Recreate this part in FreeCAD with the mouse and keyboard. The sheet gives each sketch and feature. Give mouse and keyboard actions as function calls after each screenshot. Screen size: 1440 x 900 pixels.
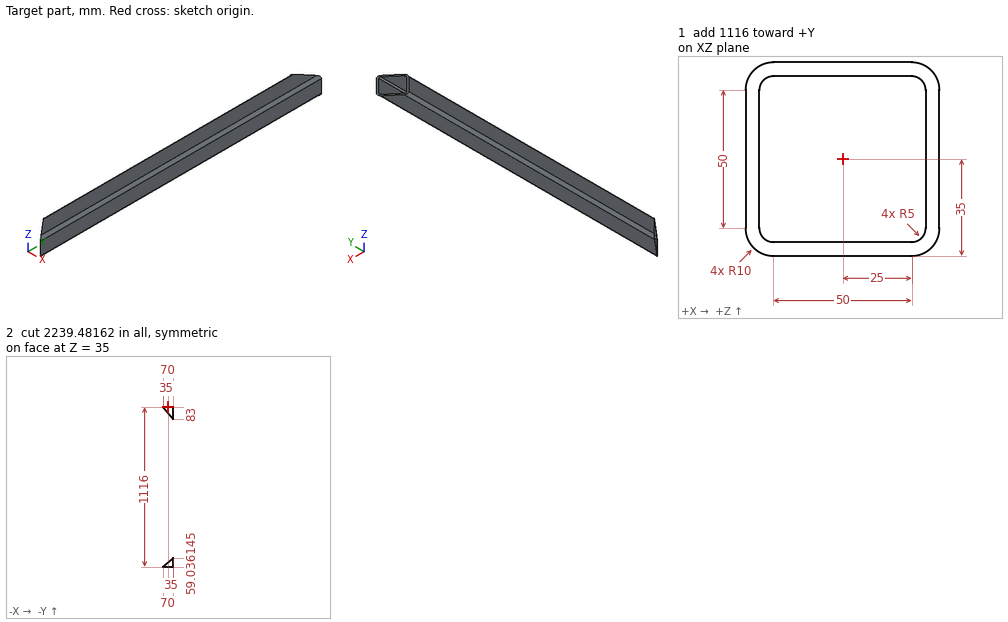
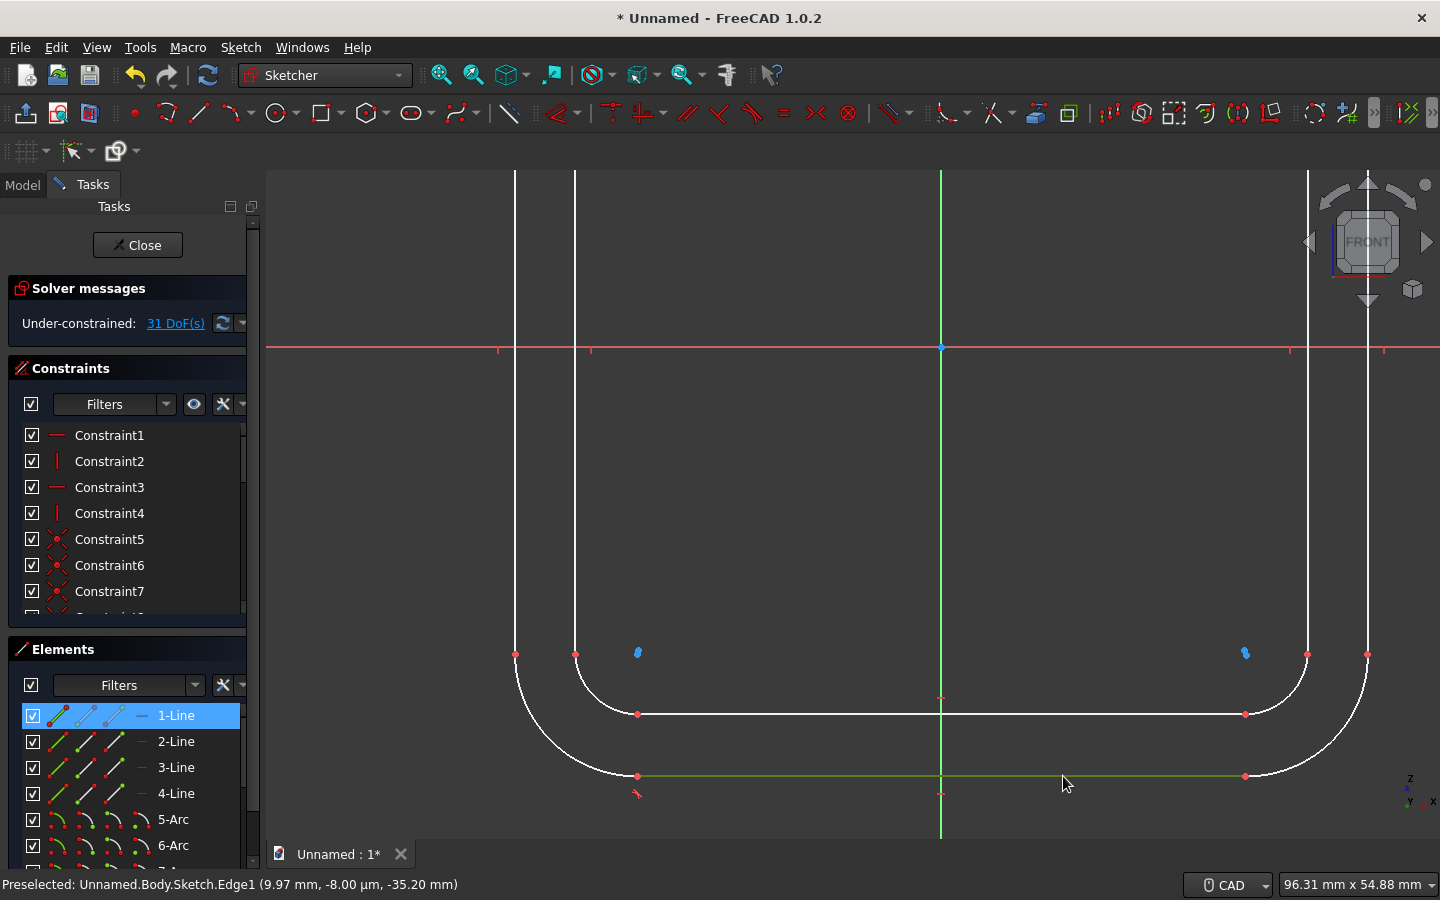
scroll(594, 696, down, 3)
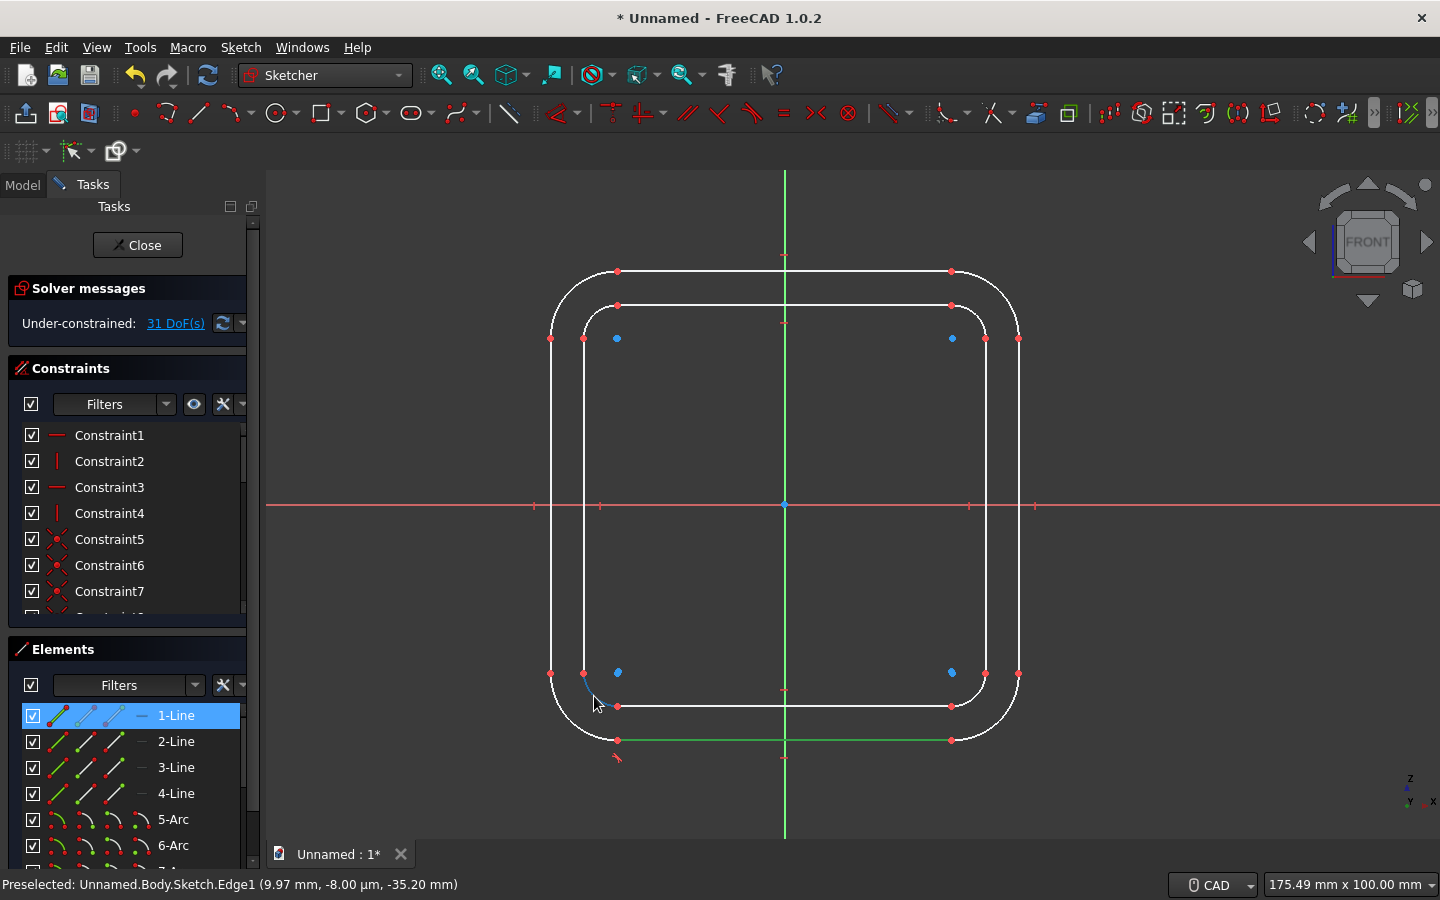
click(982, 733)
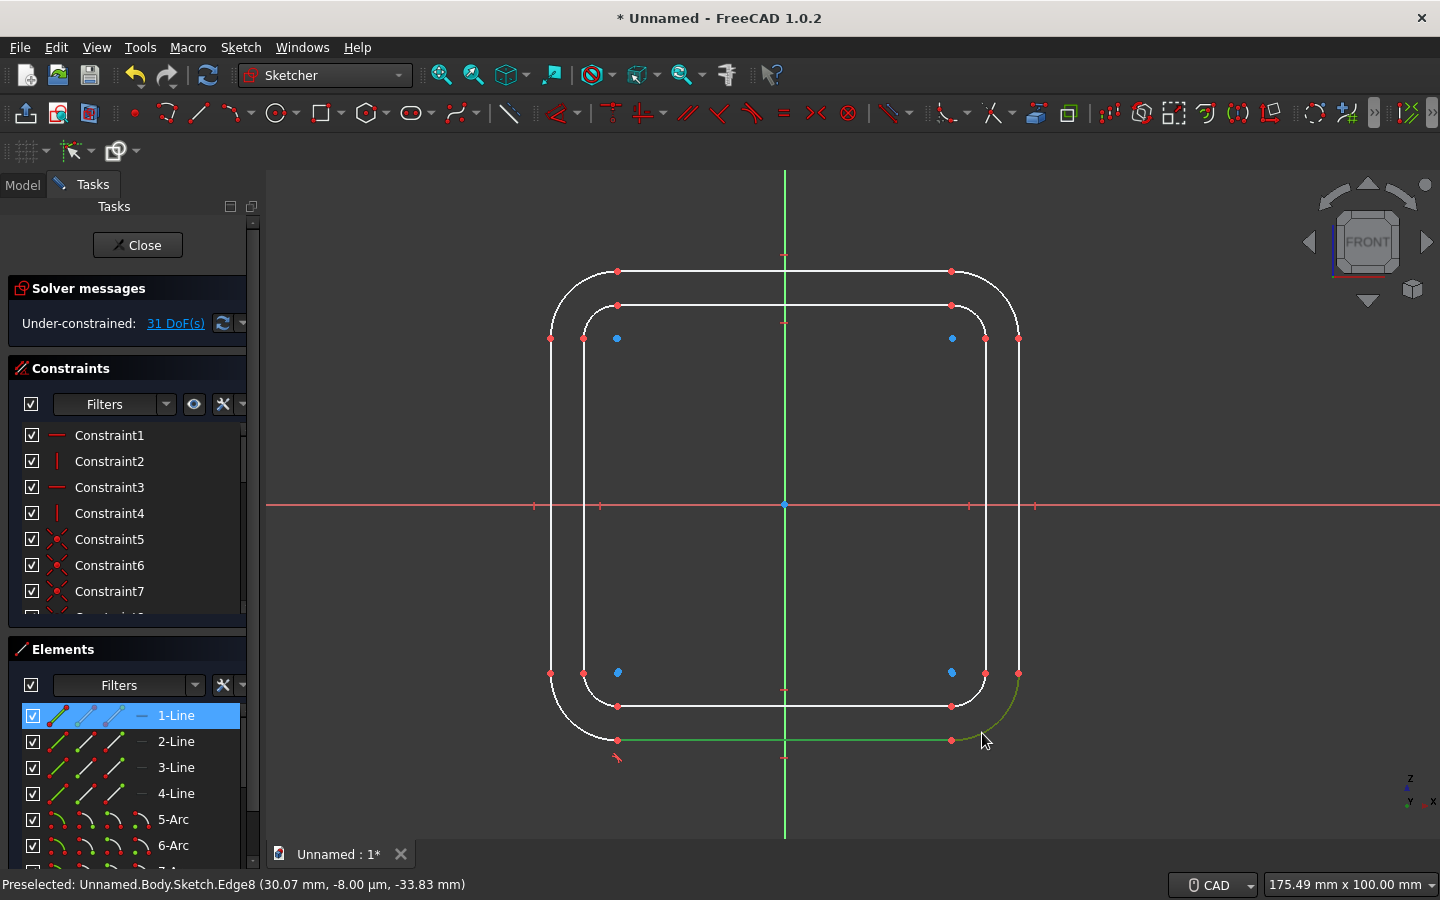
key(t)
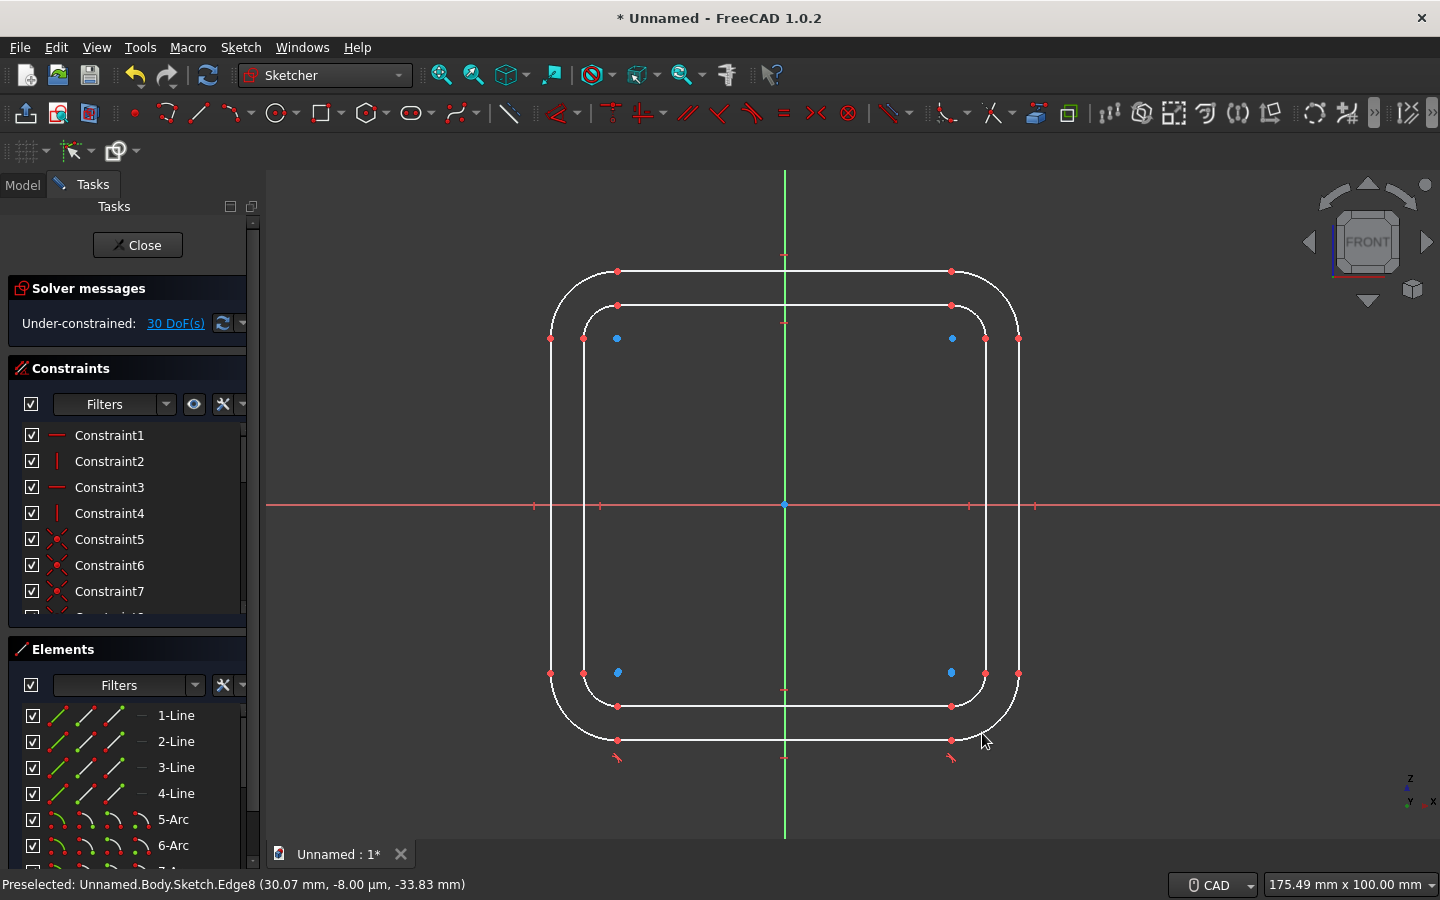
click(551, 573)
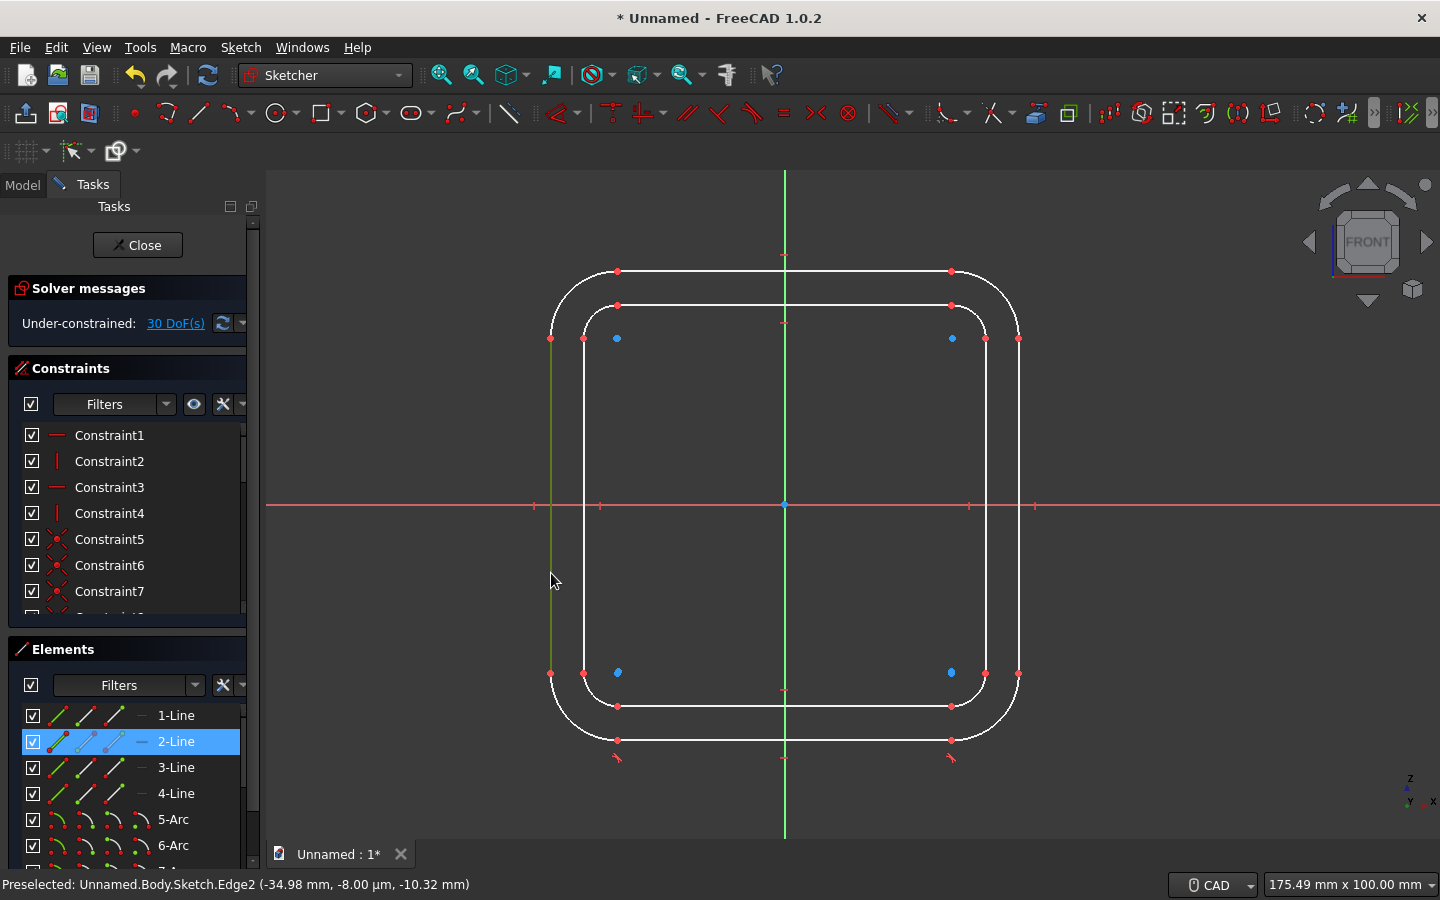
click(558, 704)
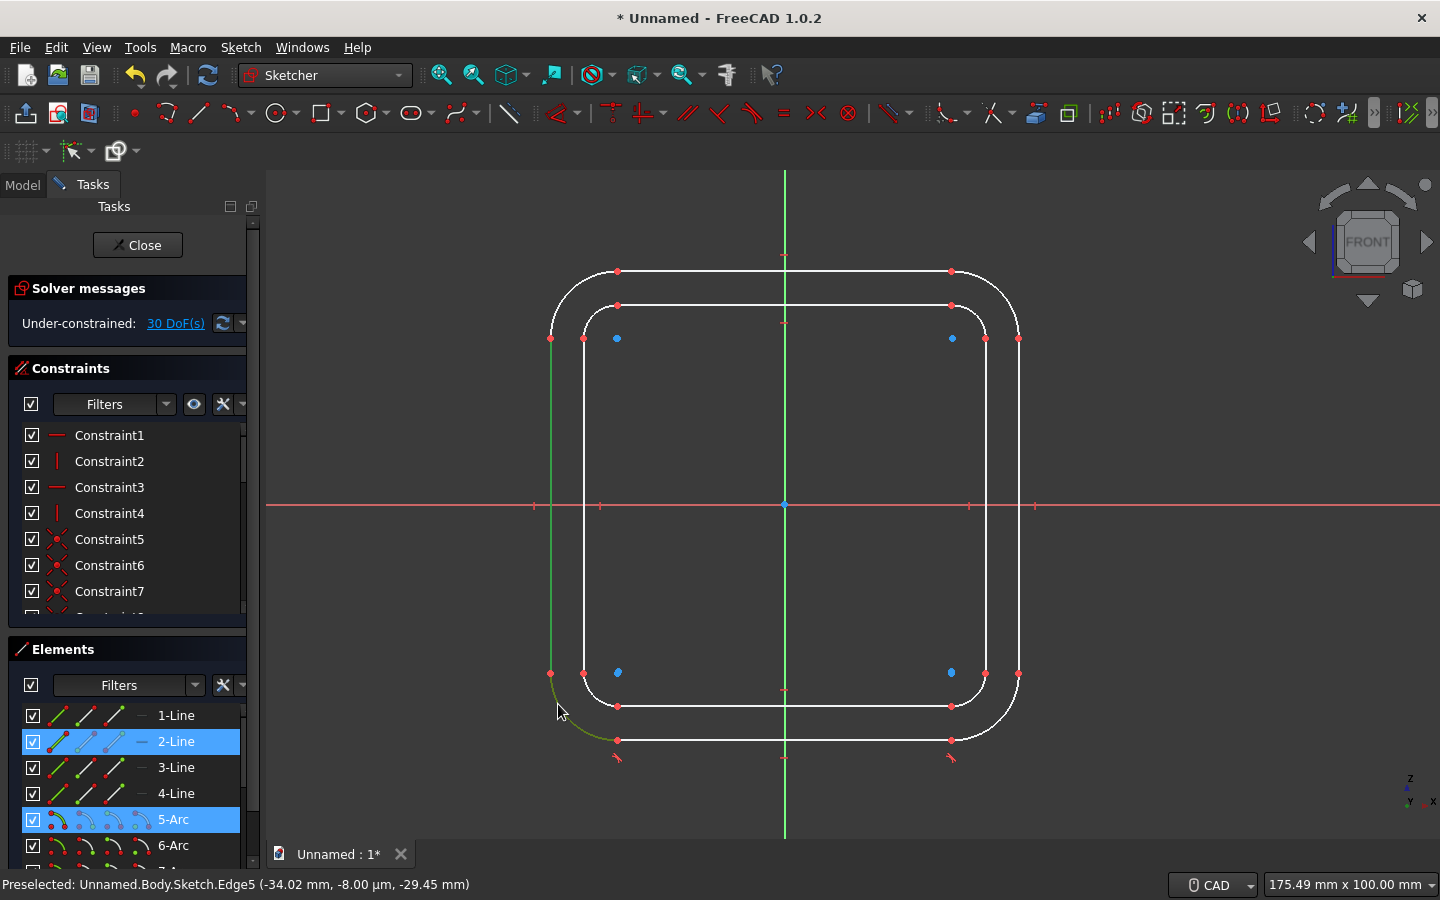
key(t)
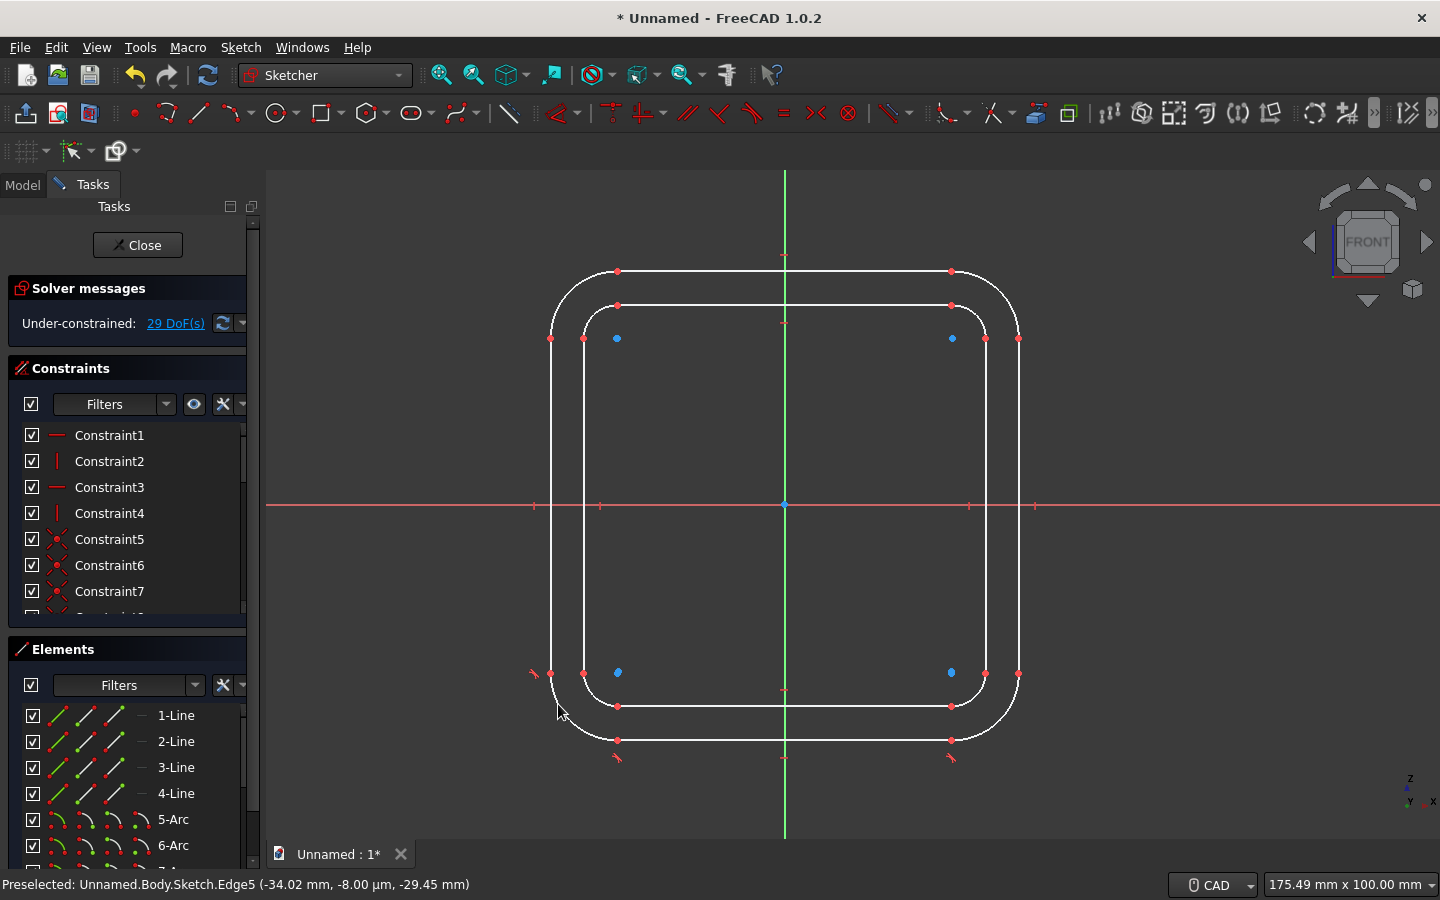
click(551, 573)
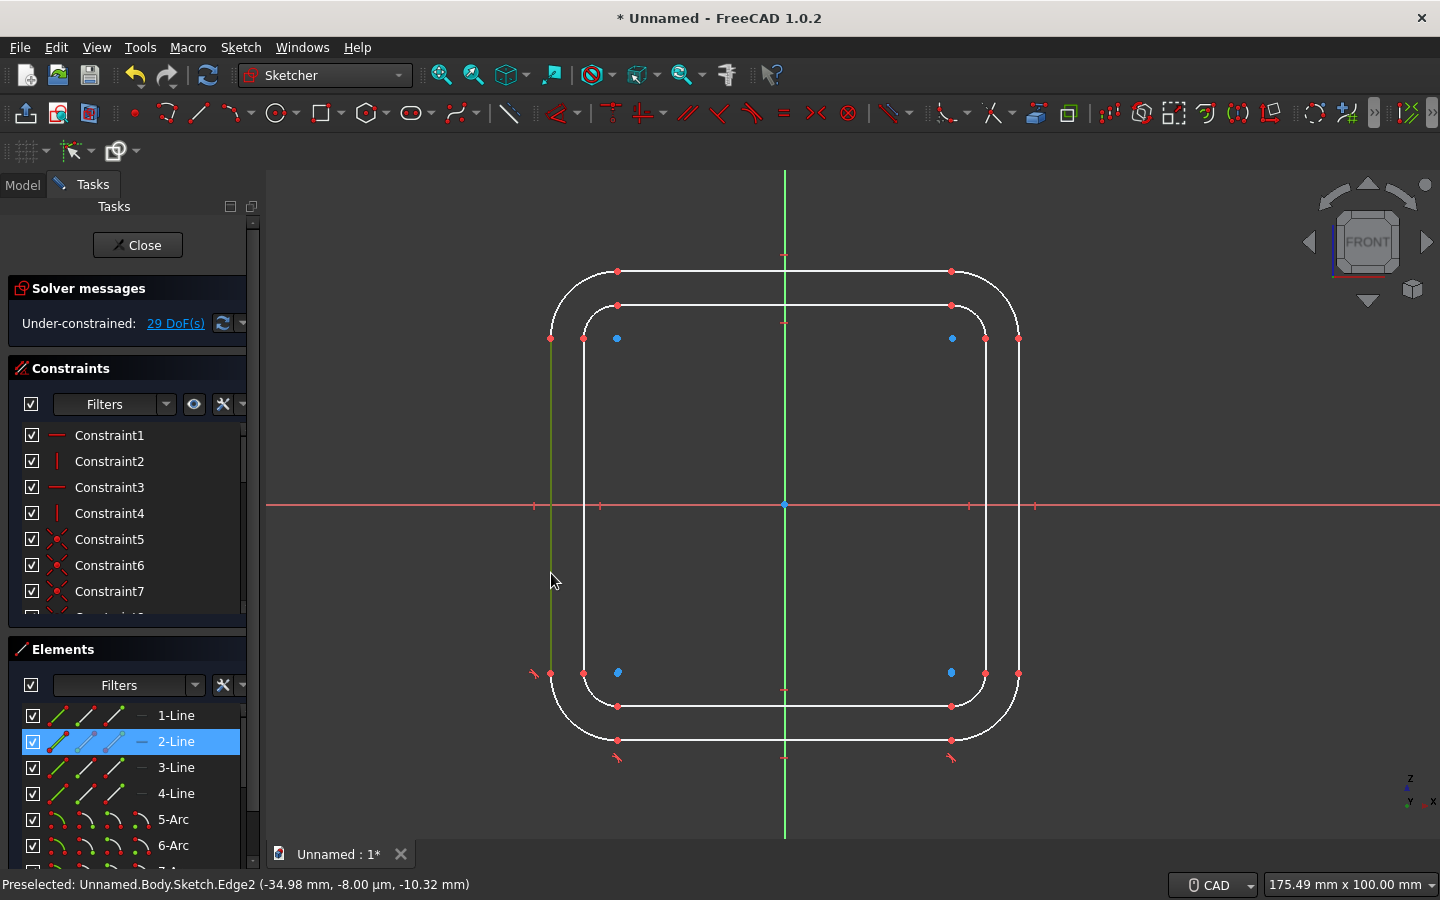
click(587, 279)